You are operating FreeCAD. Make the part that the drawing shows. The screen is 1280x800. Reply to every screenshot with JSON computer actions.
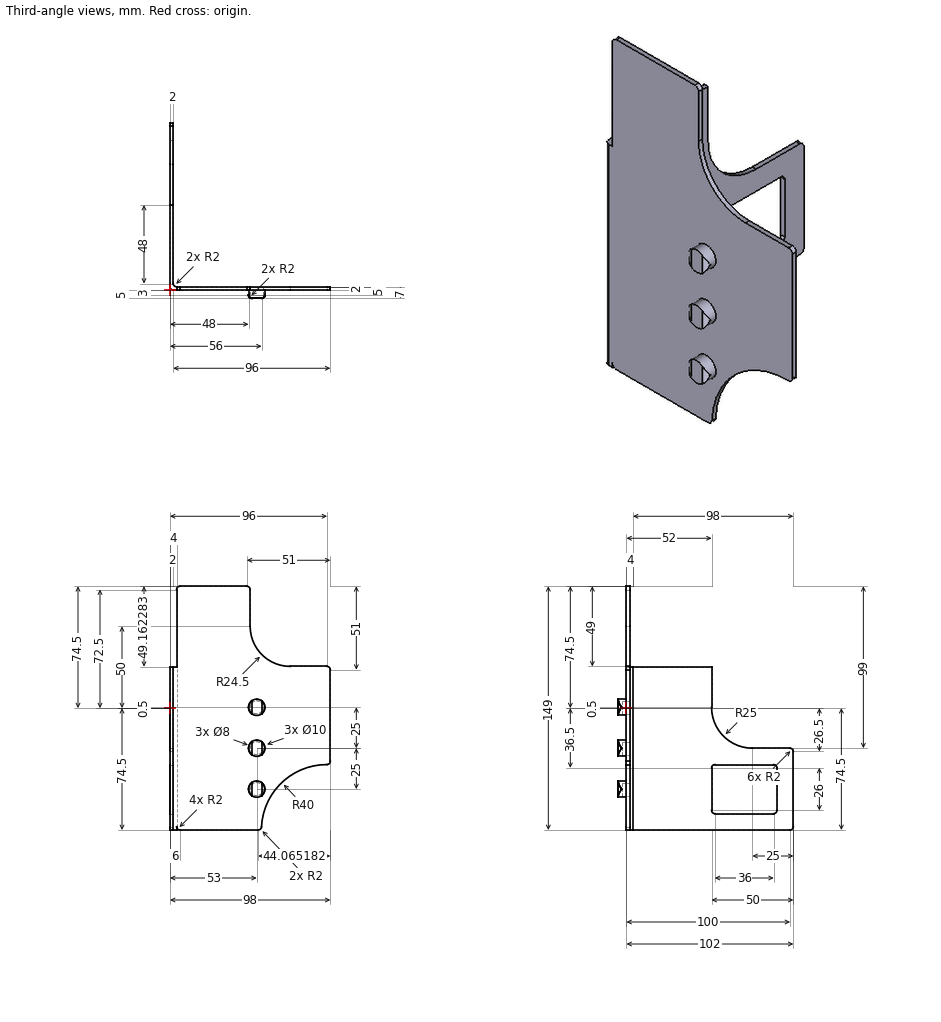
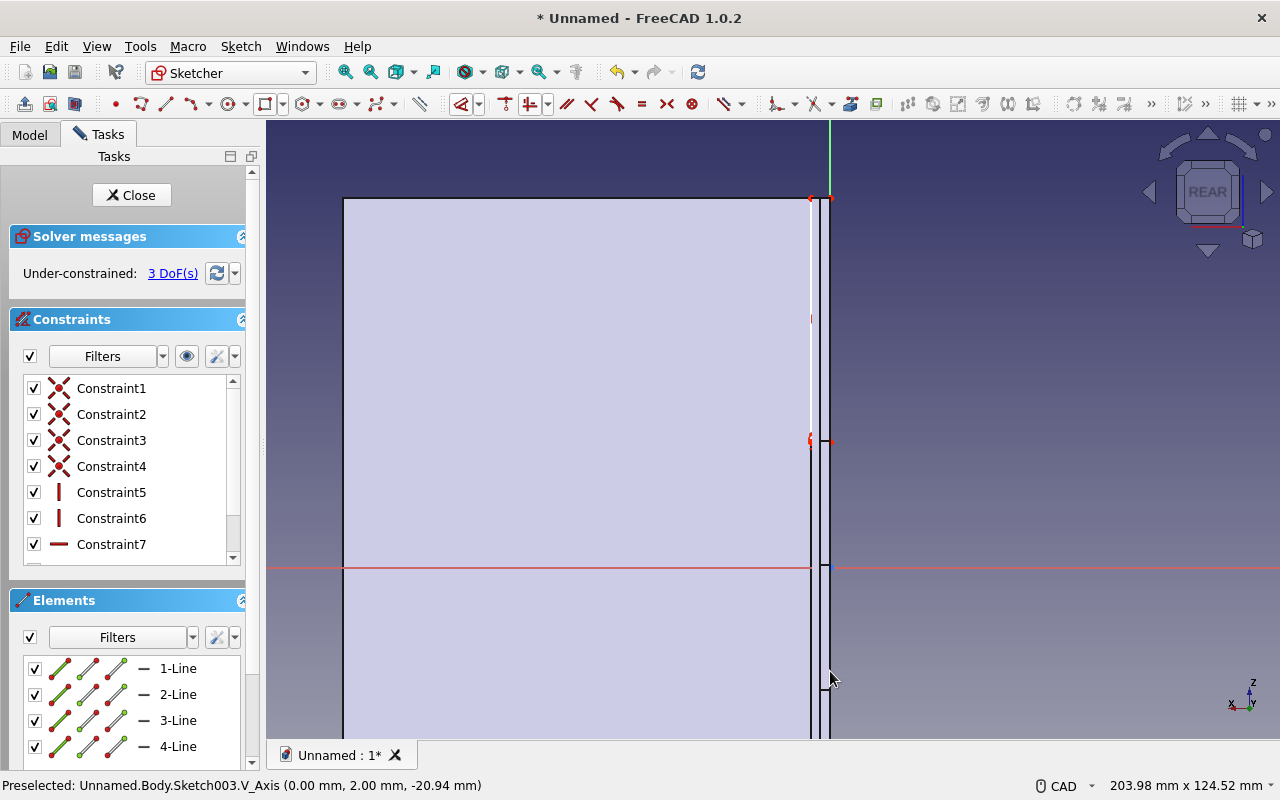
{"action": "scroll", "coordinate": [821, 443], "scroll_direction": "up", "scroll_amount": 4}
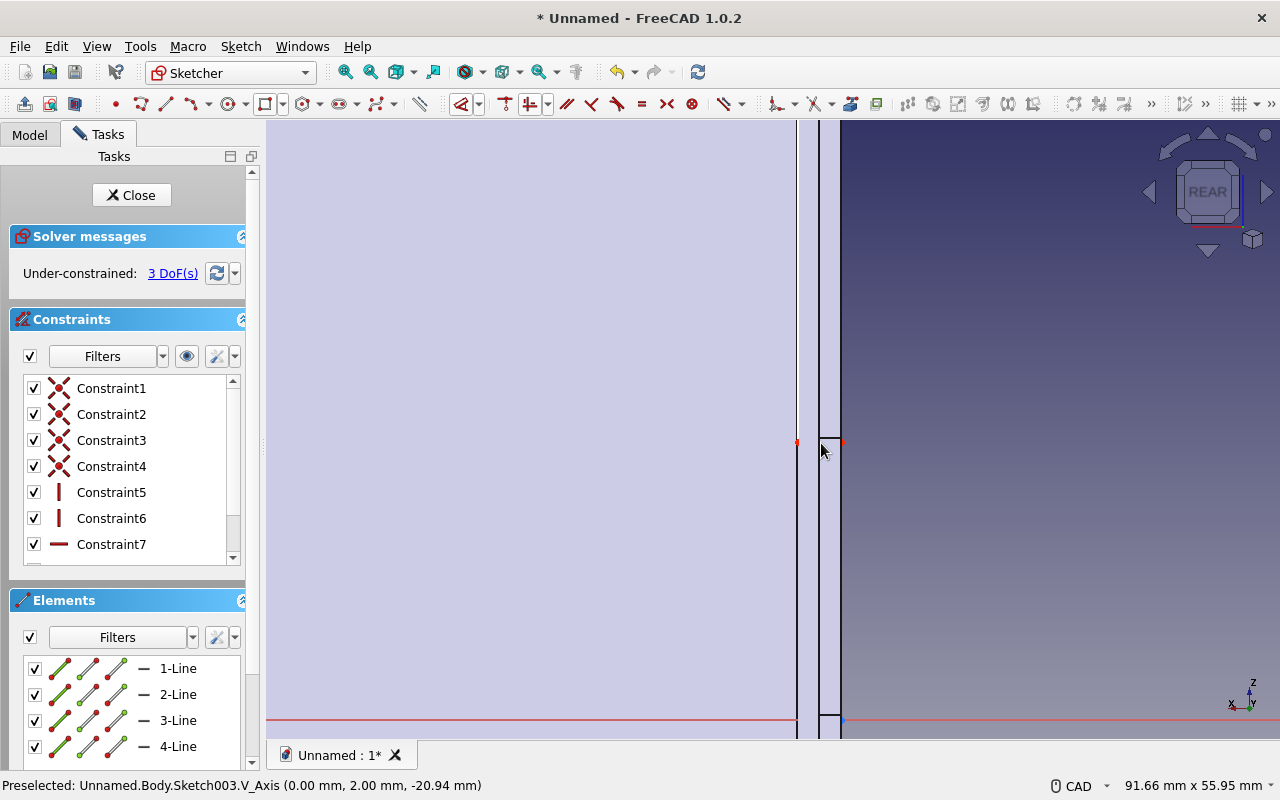
{"action": "left_click", "coordinate": [815, 442]}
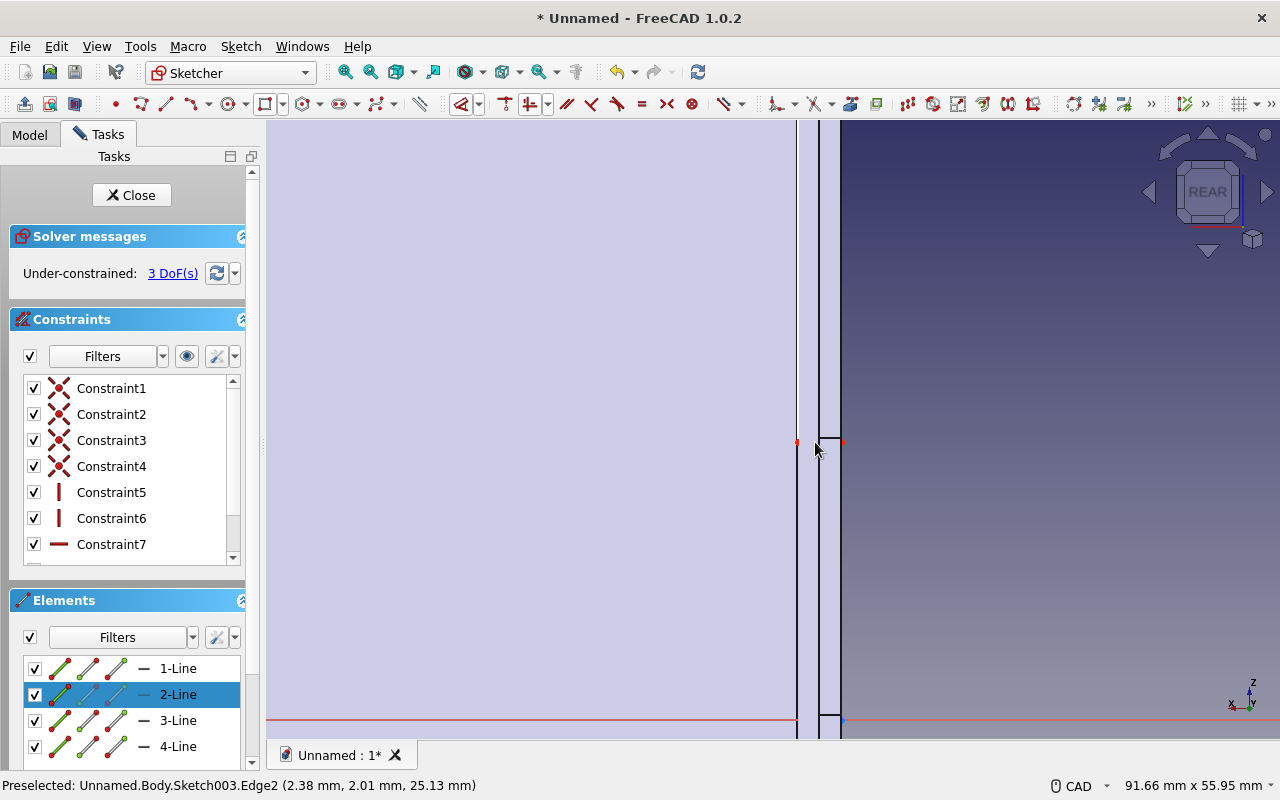
{"action": "key", "text": "l"}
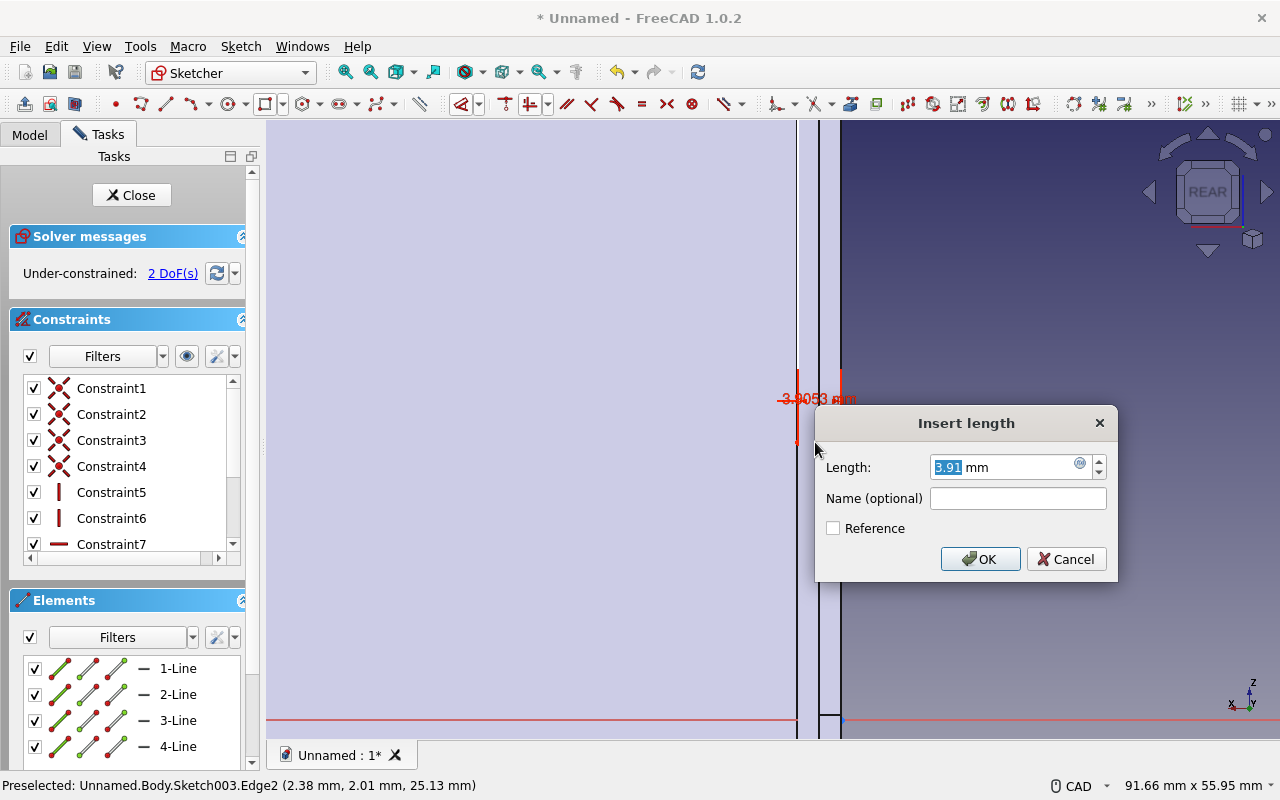
{"action": "type", "text": "4"}
{"action": "key", "text": "Return"}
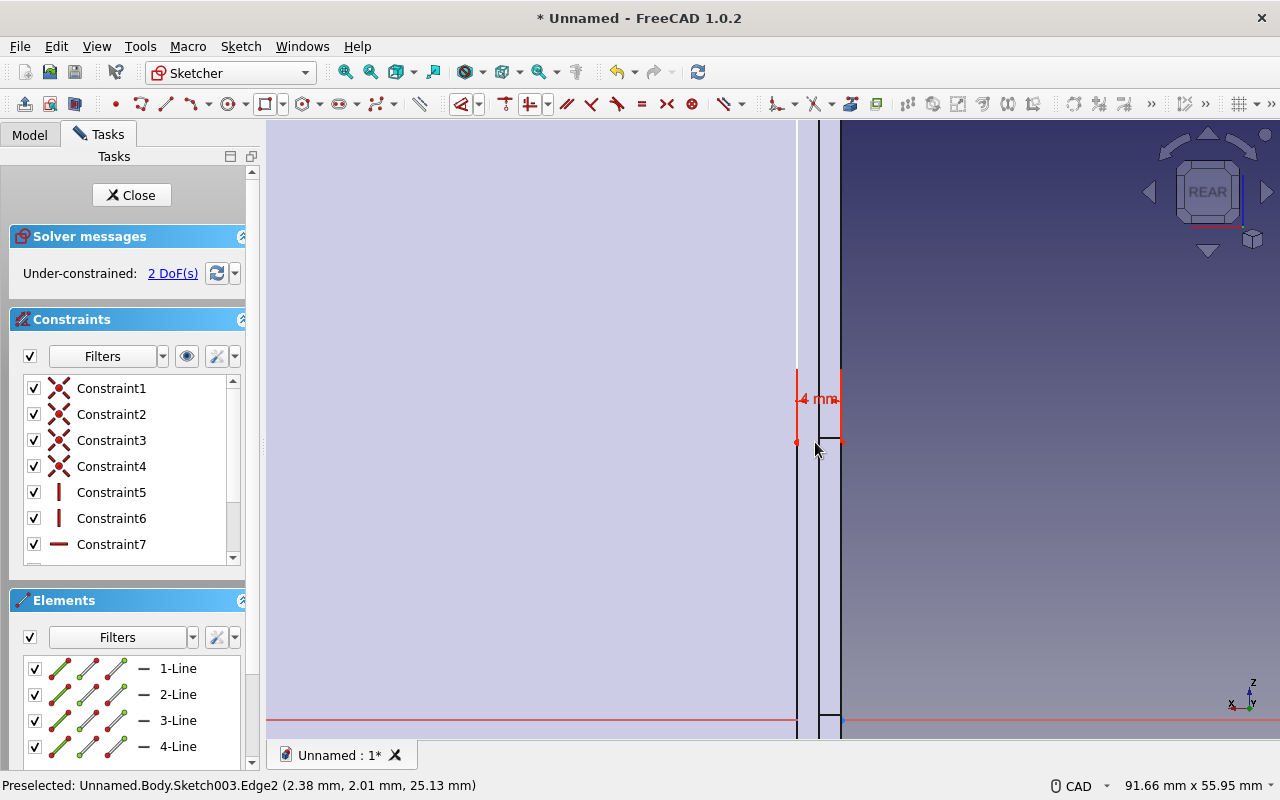
{"action": "scroll", "coordinate": [611, 528], "scroll_direction": "down", "scroll_amount": 4}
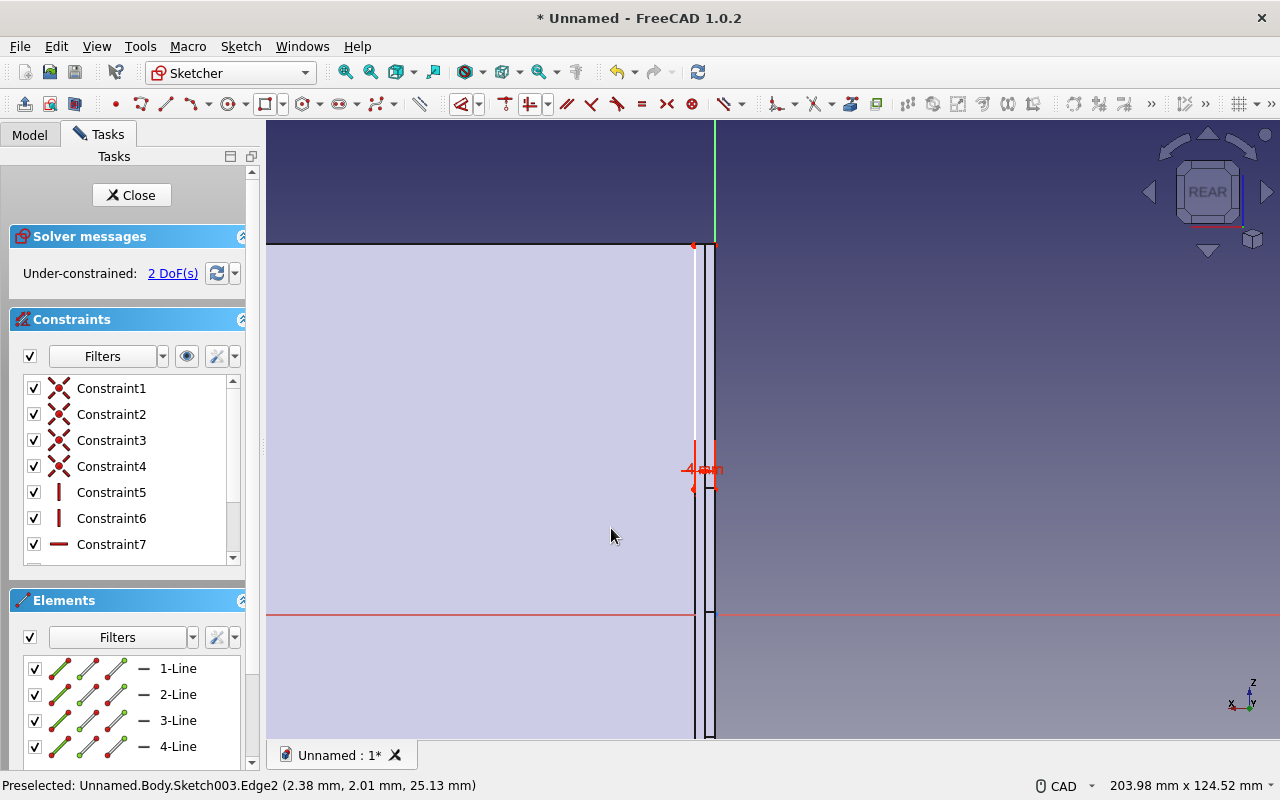
{"action": "left_click", "coordinate": [695, 246]}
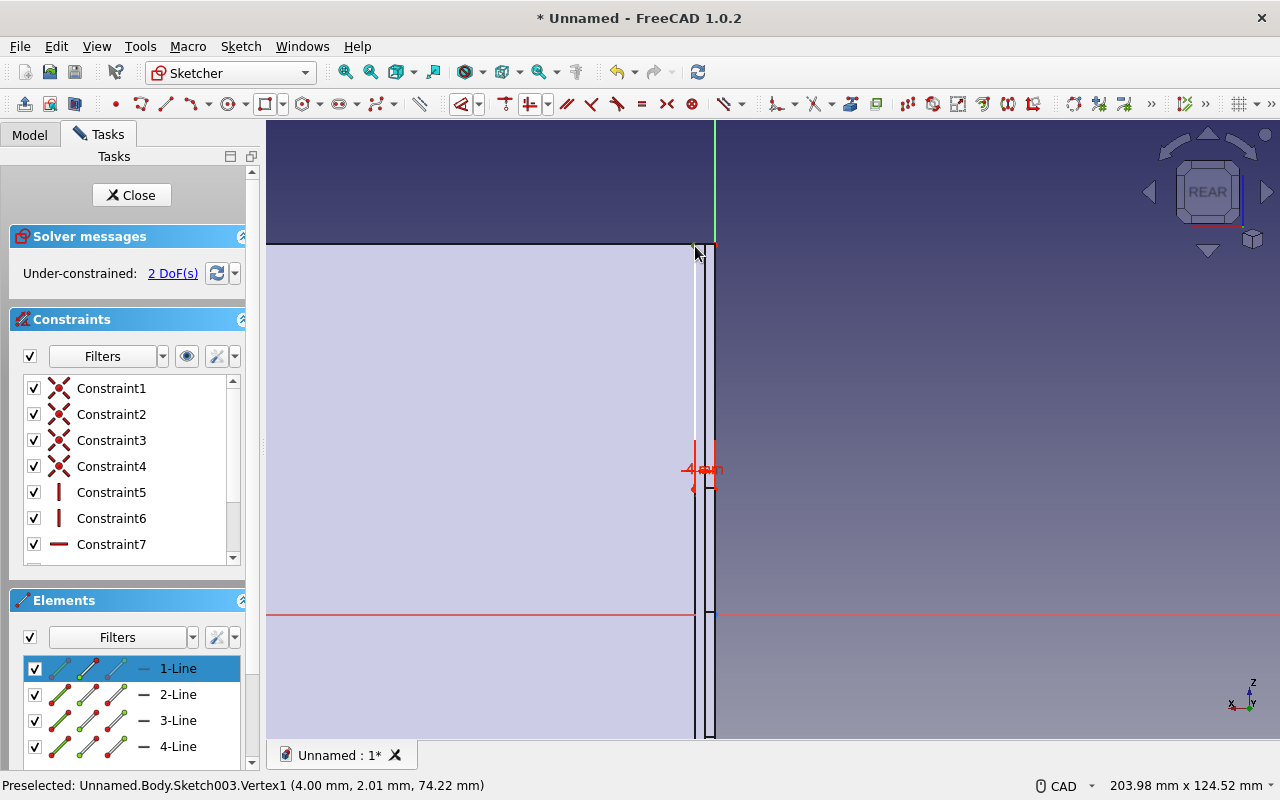
{"action": "key", "text": "i"}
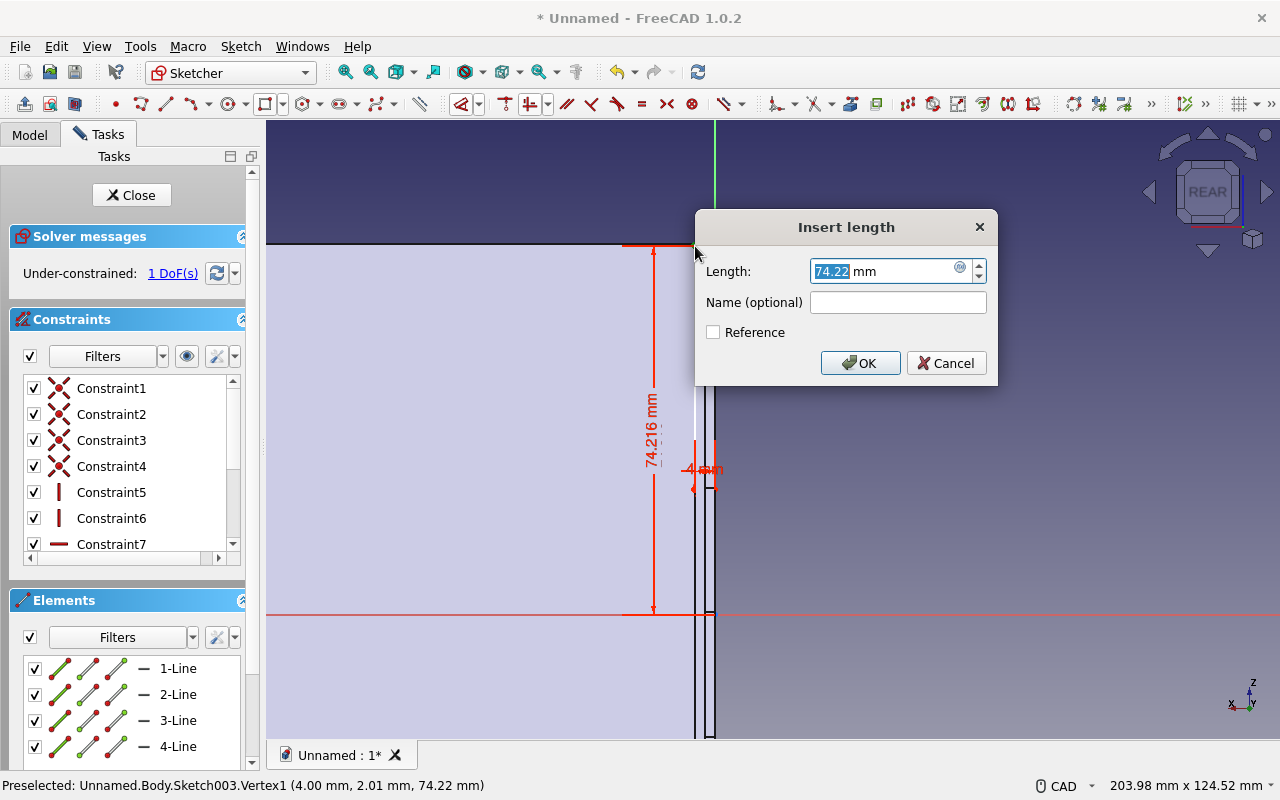
{"action": "type", "text": "74.5"}
{"action": "key", "text": "Return"}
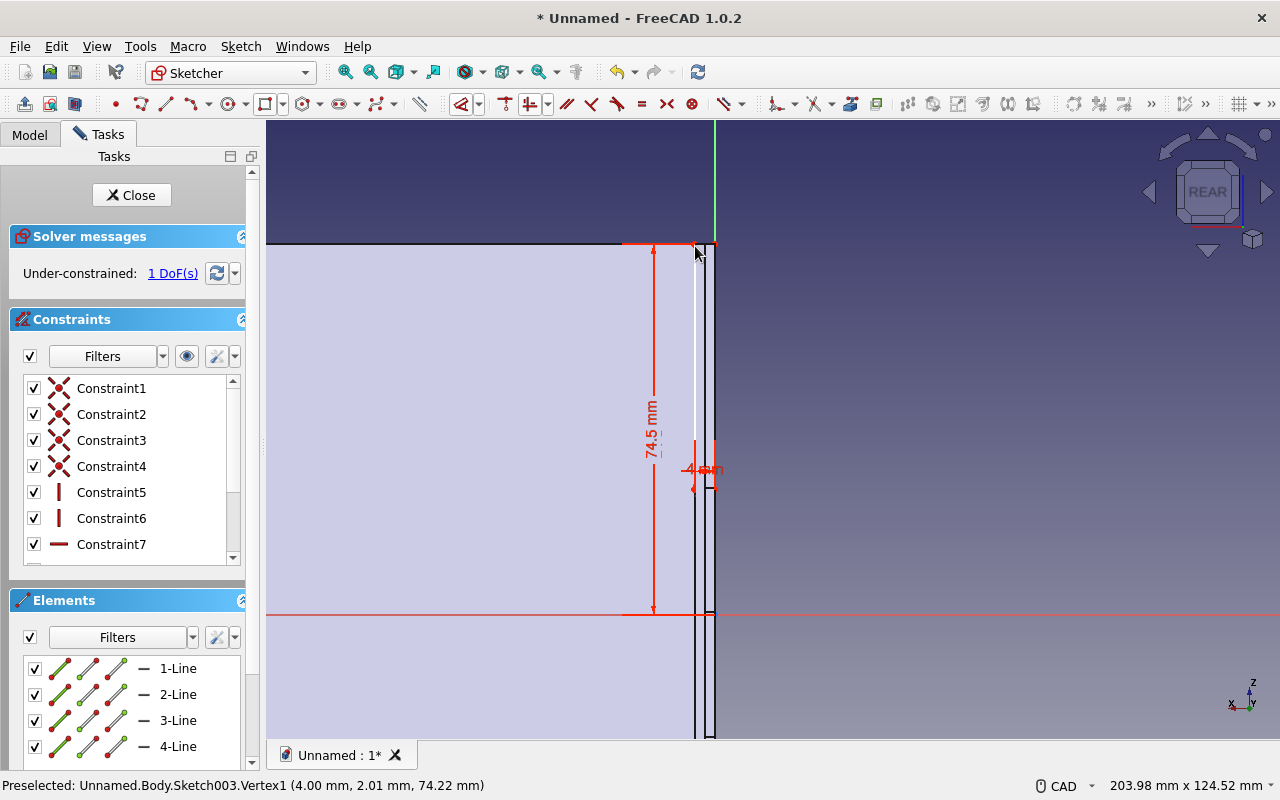
{"action": "left_click", "coordinate": [695, 318]}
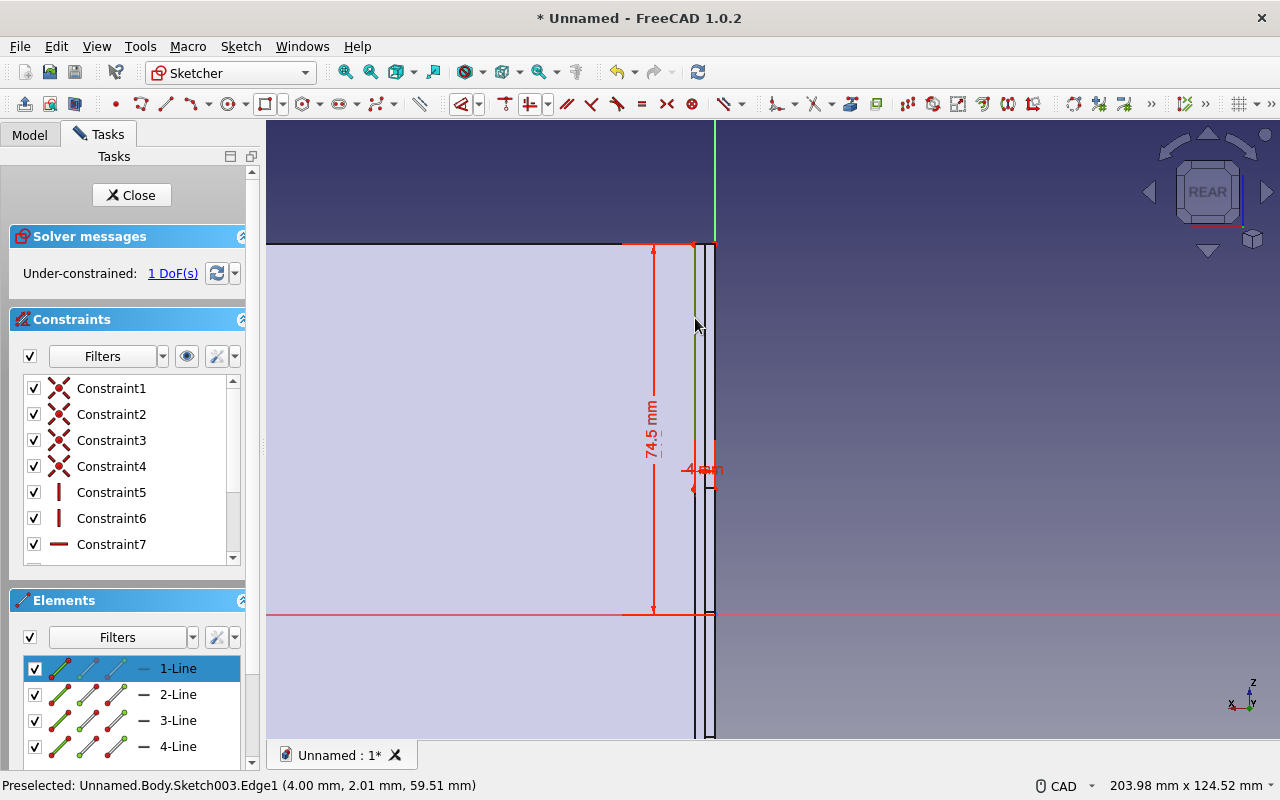
{"action": "key", "text": "i"}